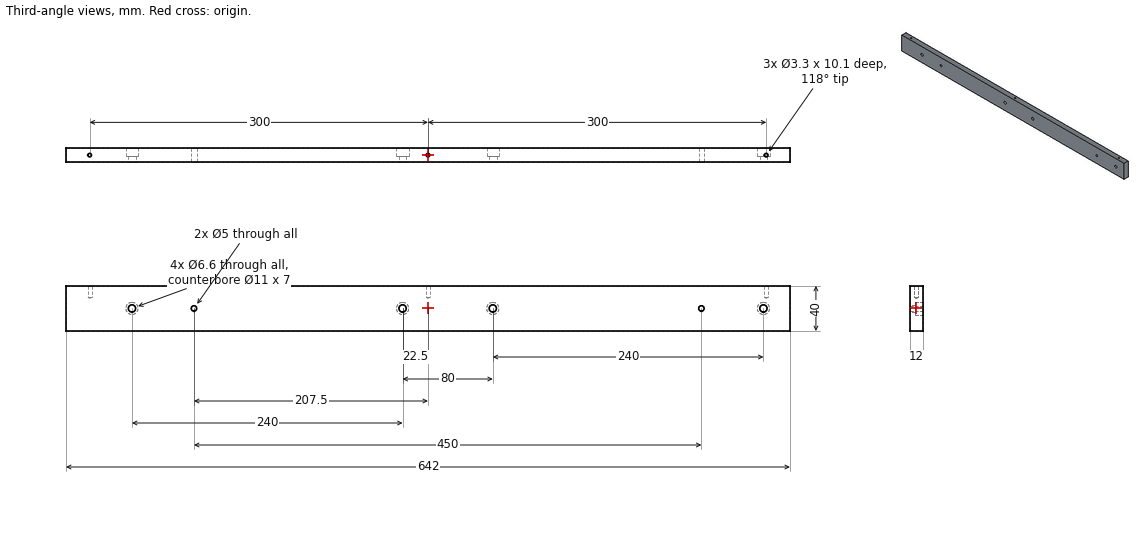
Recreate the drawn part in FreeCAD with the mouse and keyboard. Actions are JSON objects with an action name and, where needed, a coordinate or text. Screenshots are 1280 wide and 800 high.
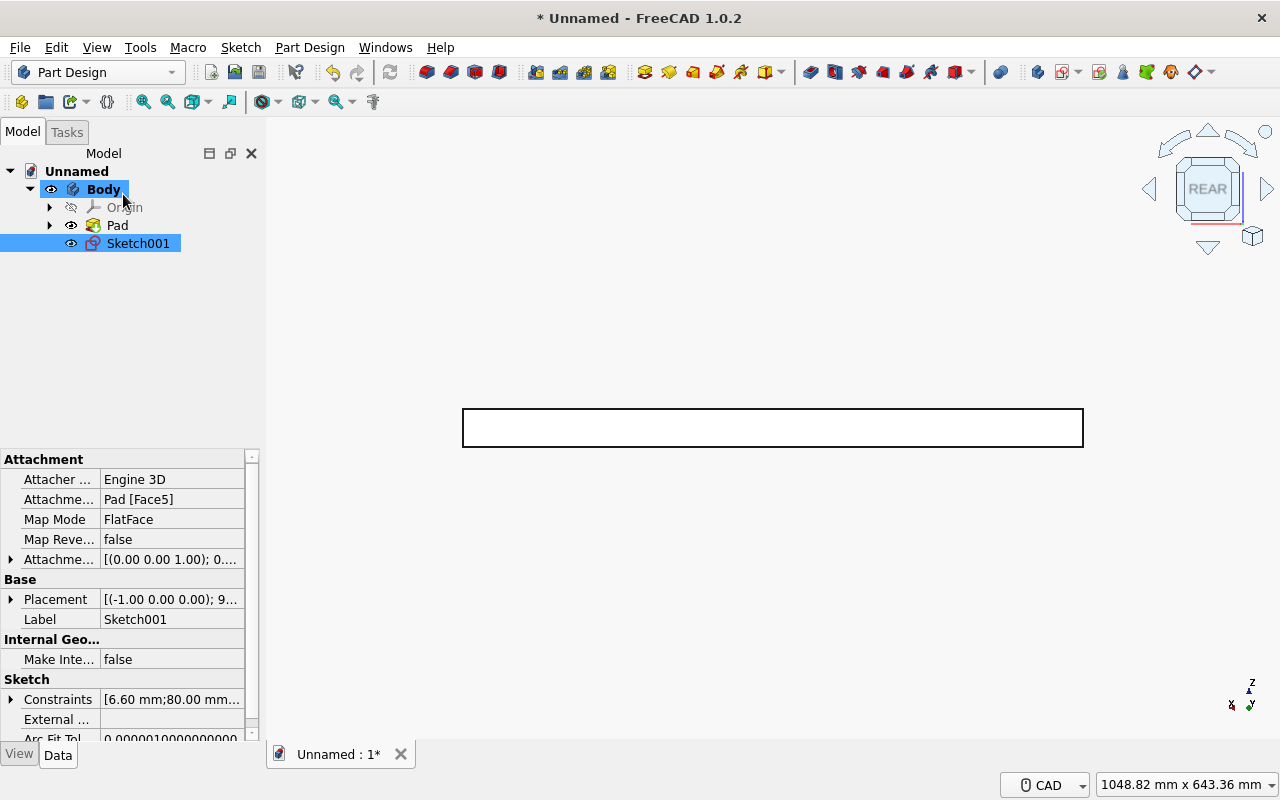
{"action": "left_click", "coordinate": [836, 72]}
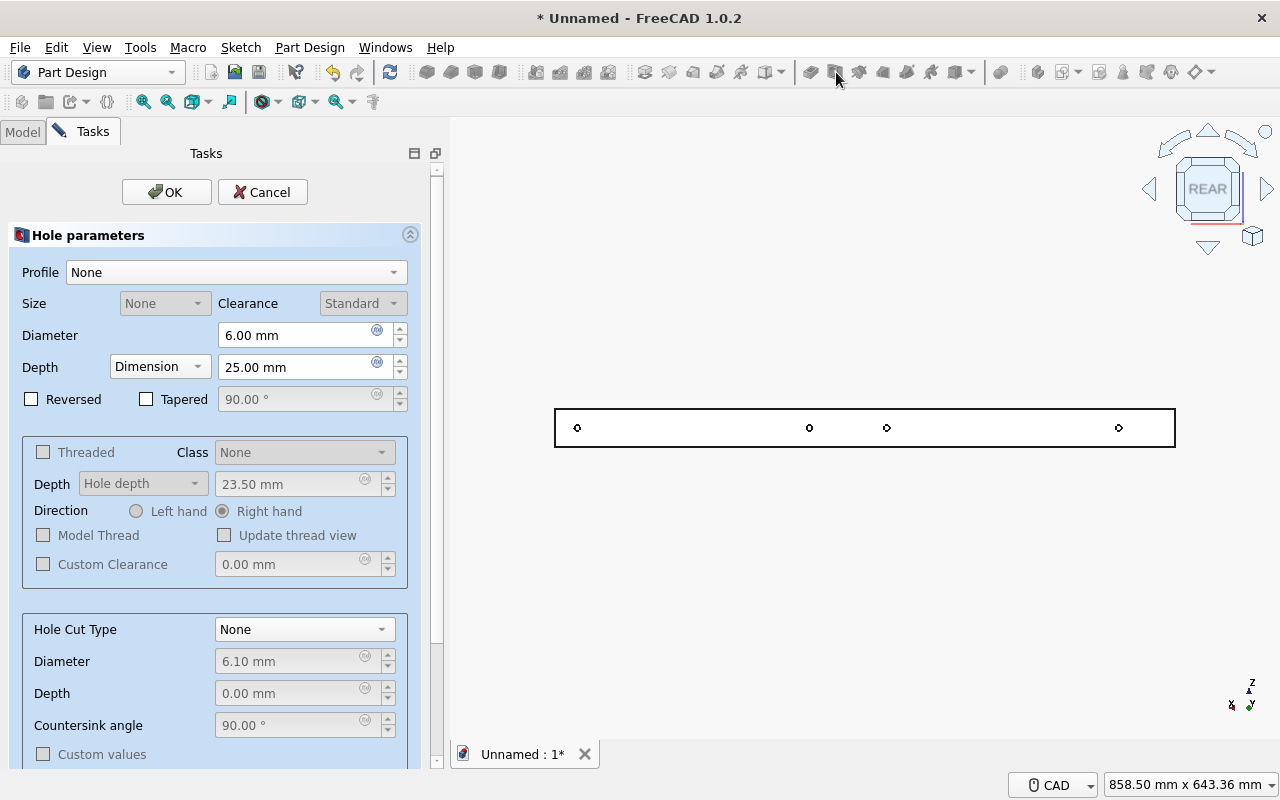
{"action": "triple_click", "coordinate": [305, 335]}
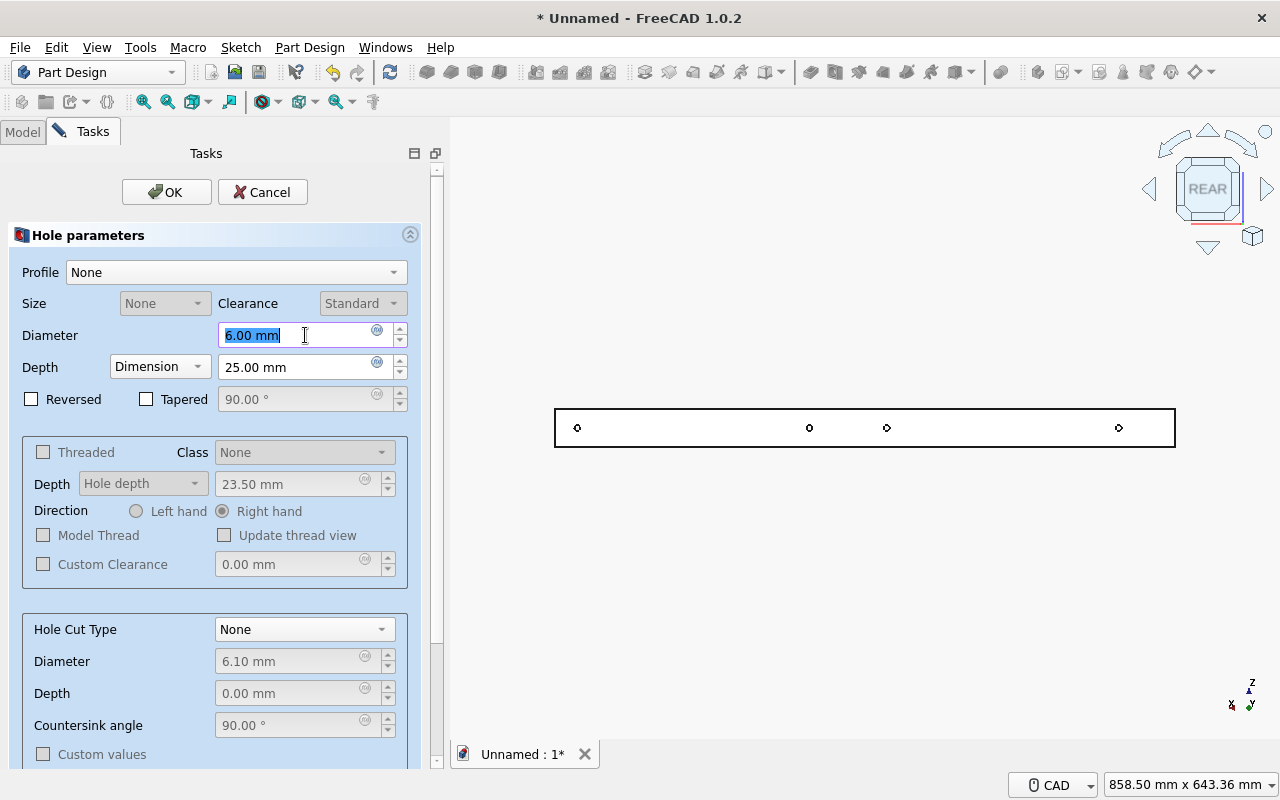
{"action": "type", "text": "6.6"}
{"action": "key", "text": "Tab"}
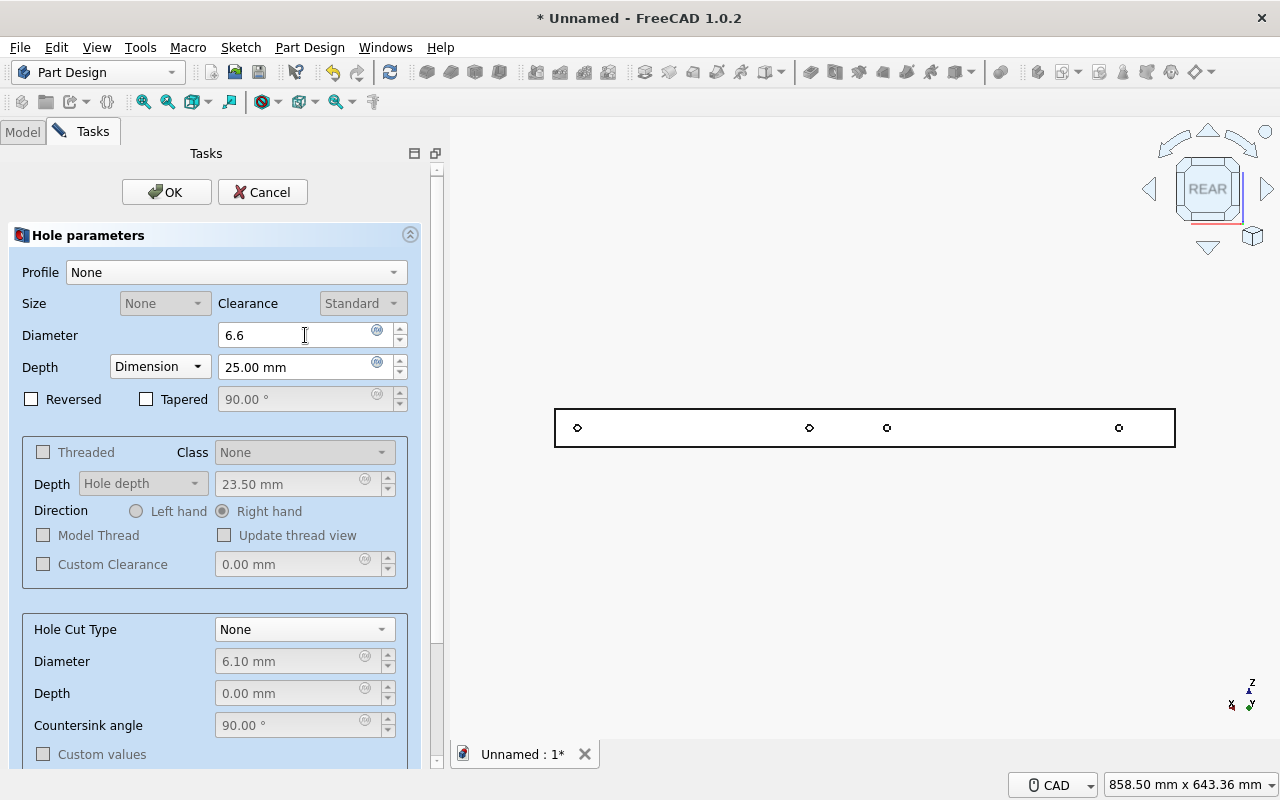
{"action": "left_click", "coordinate": [161, 366]}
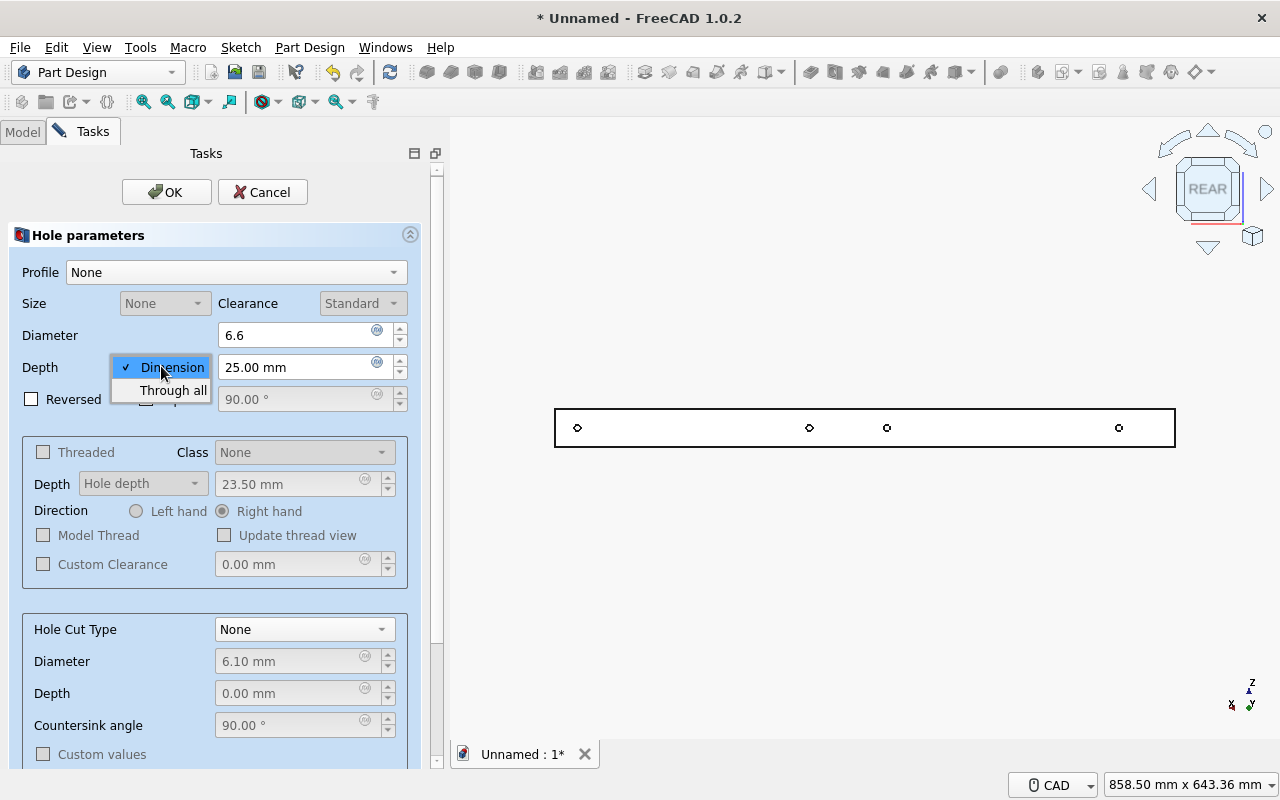
{"action": "left_click", "coordinate": [160, 390]}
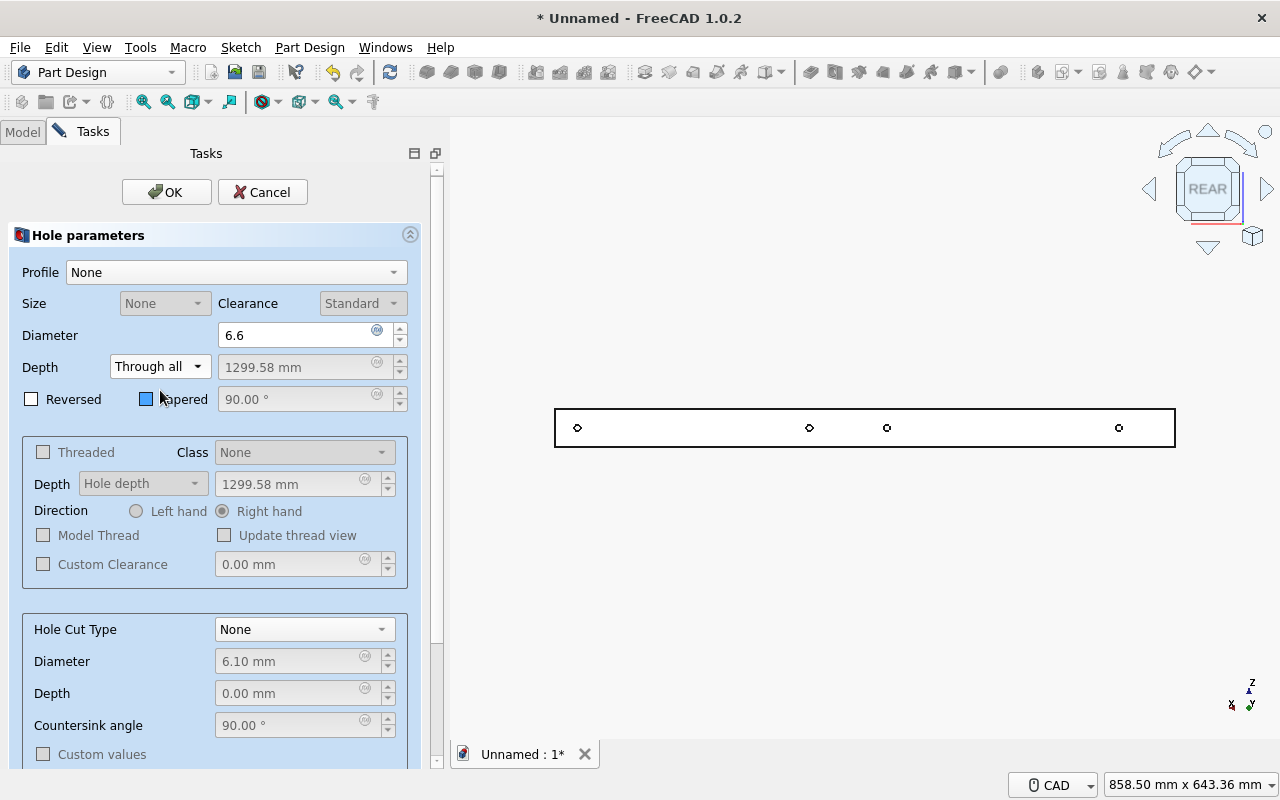
{"action": "left_click", "coordinate": [306, 630]}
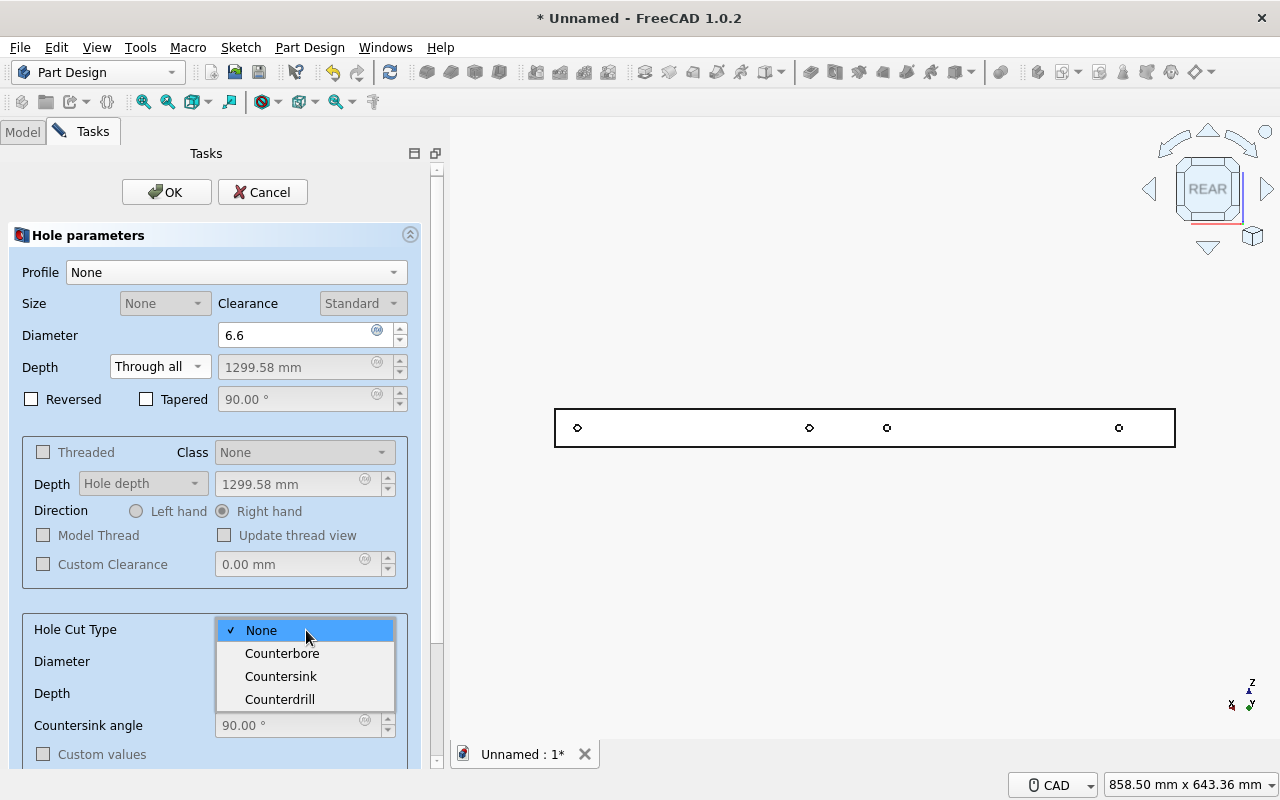
{"action": "left_click", "coordinate": [304, 654]}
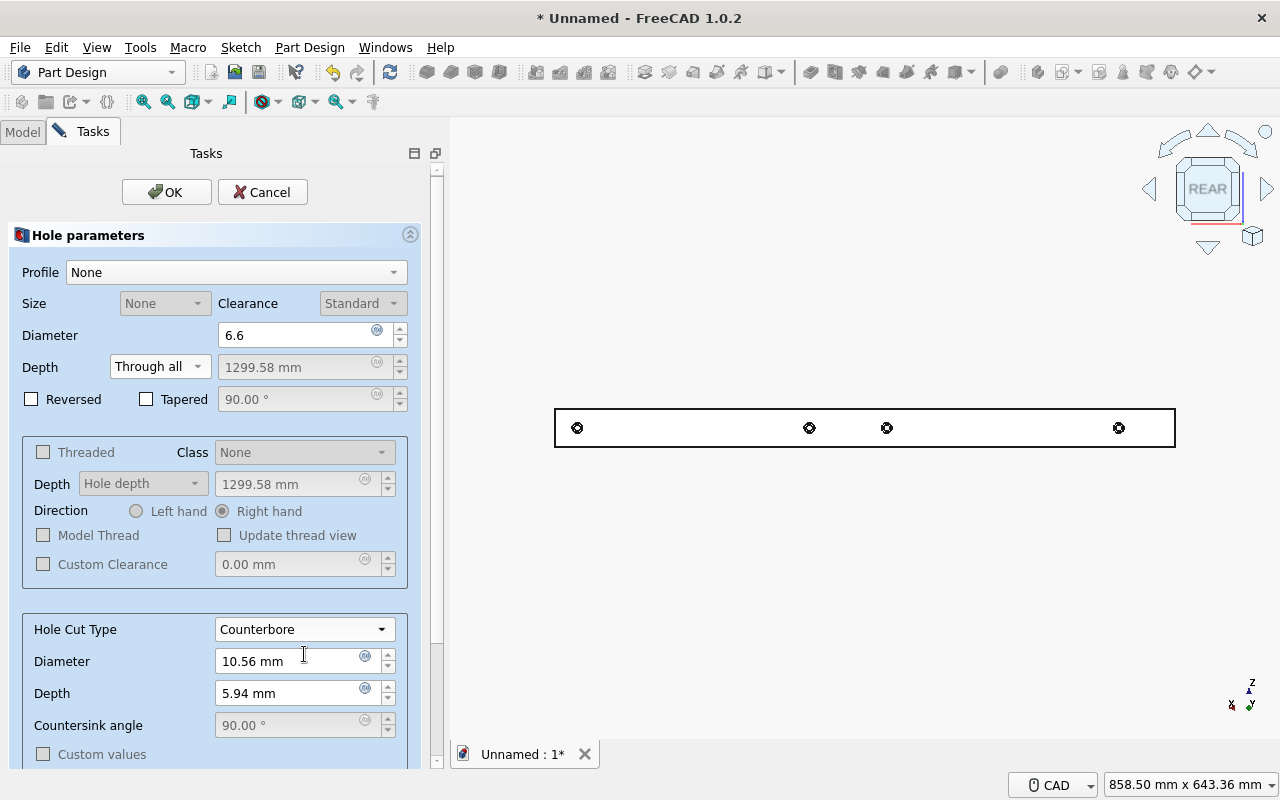
{"action": "triple_click", "coordinate": [298, 661]}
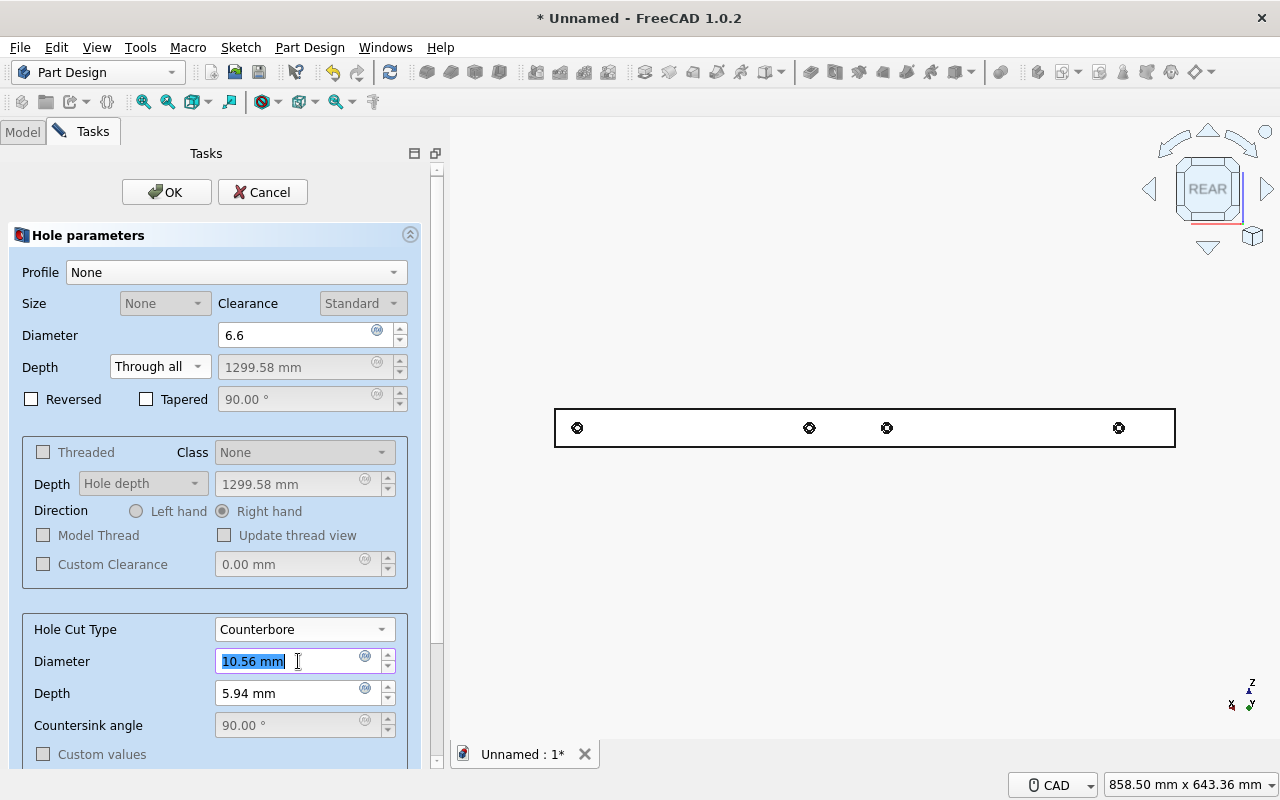
{"action": "type", "text": "11"}
{"action": "key", "text": "Tab"}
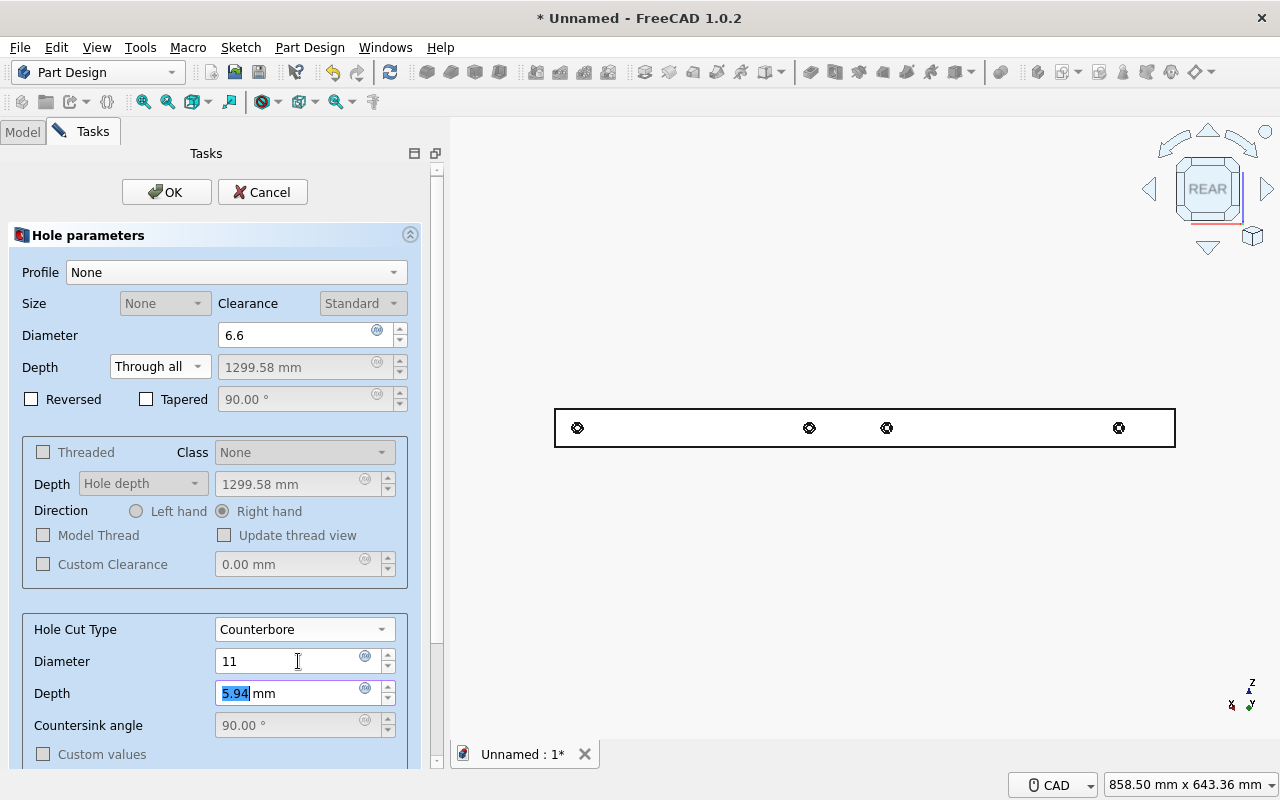
{"action": "type", "text": "7"}
{"action": "key", "text": "Tab"}